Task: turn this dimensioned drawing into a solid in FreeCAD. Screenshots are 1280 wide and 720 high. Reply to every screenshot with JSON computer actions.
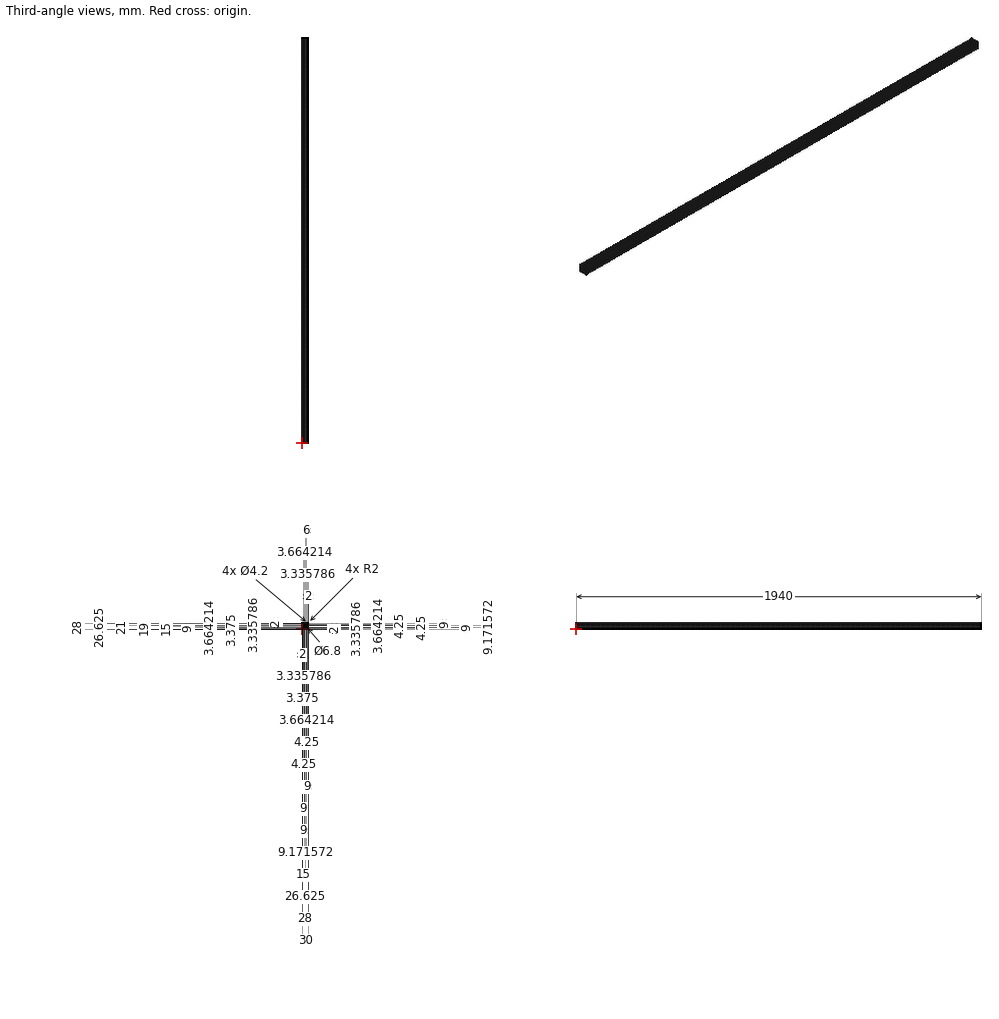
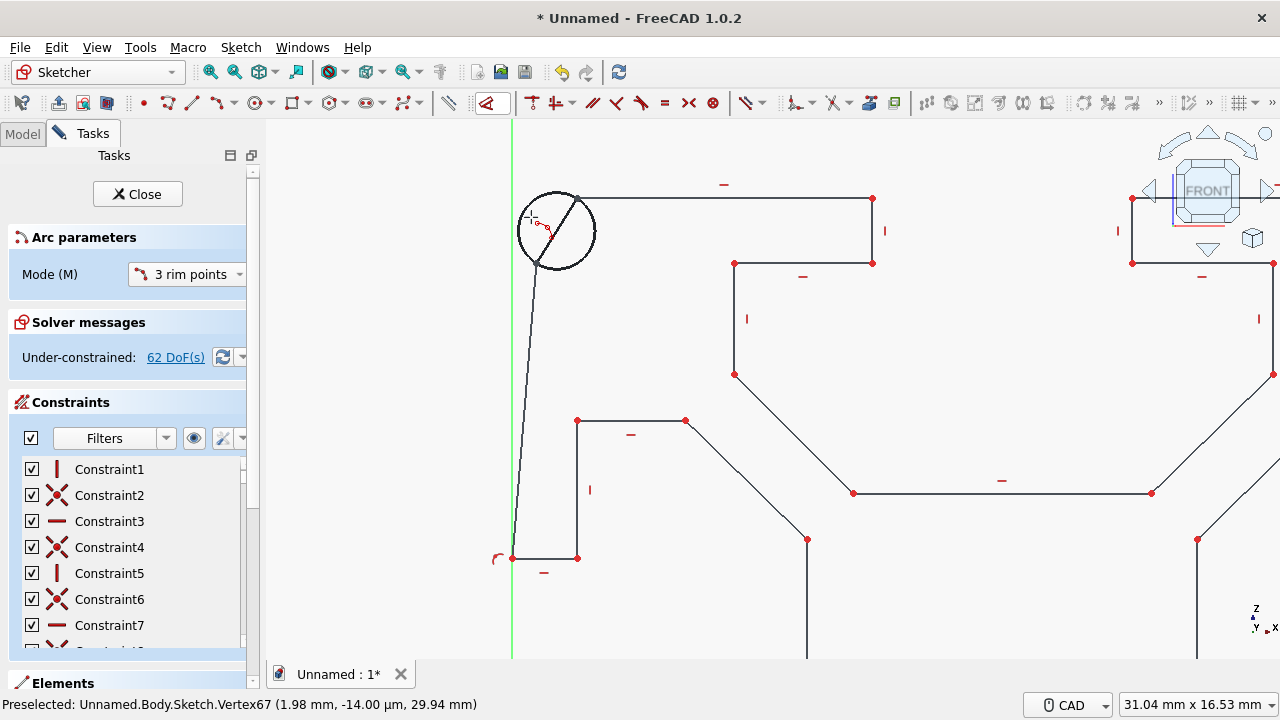
{"action": "left_click", "coordinate": [532, 216]}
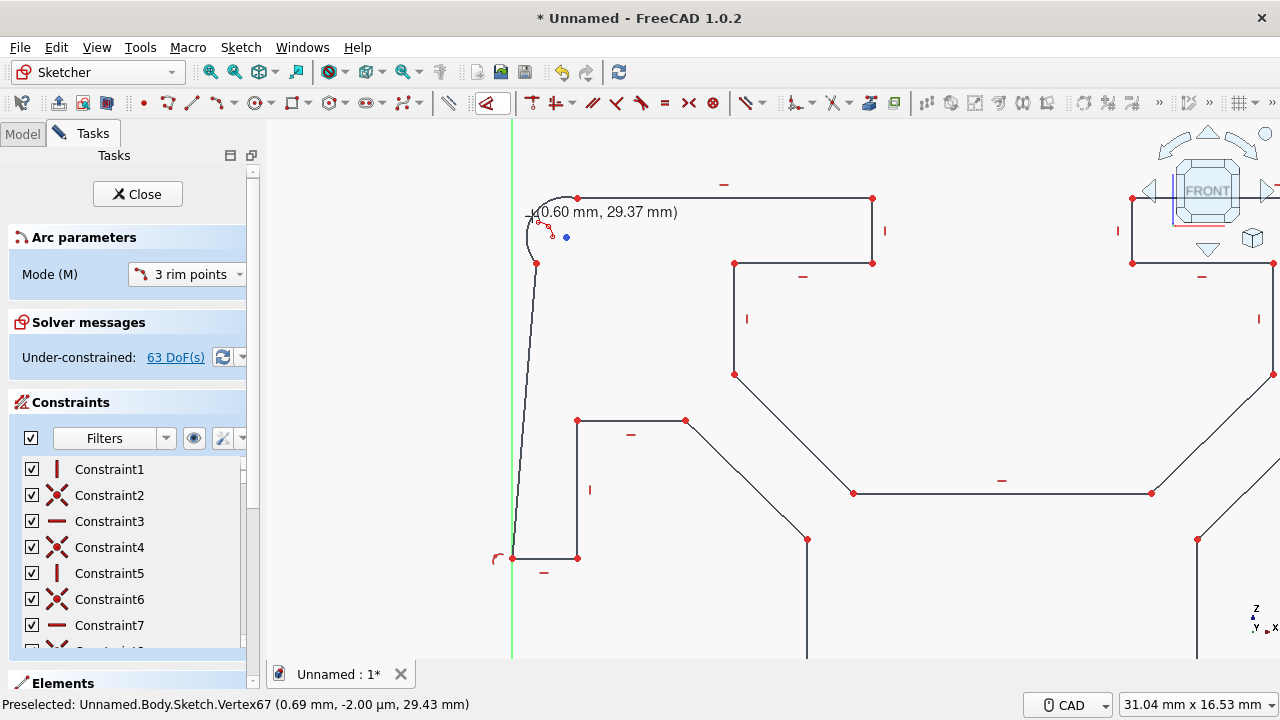
{"action": "scroll", "coordinate": [531, 216], "scroll_direction": "down", "scroll_amount": 5}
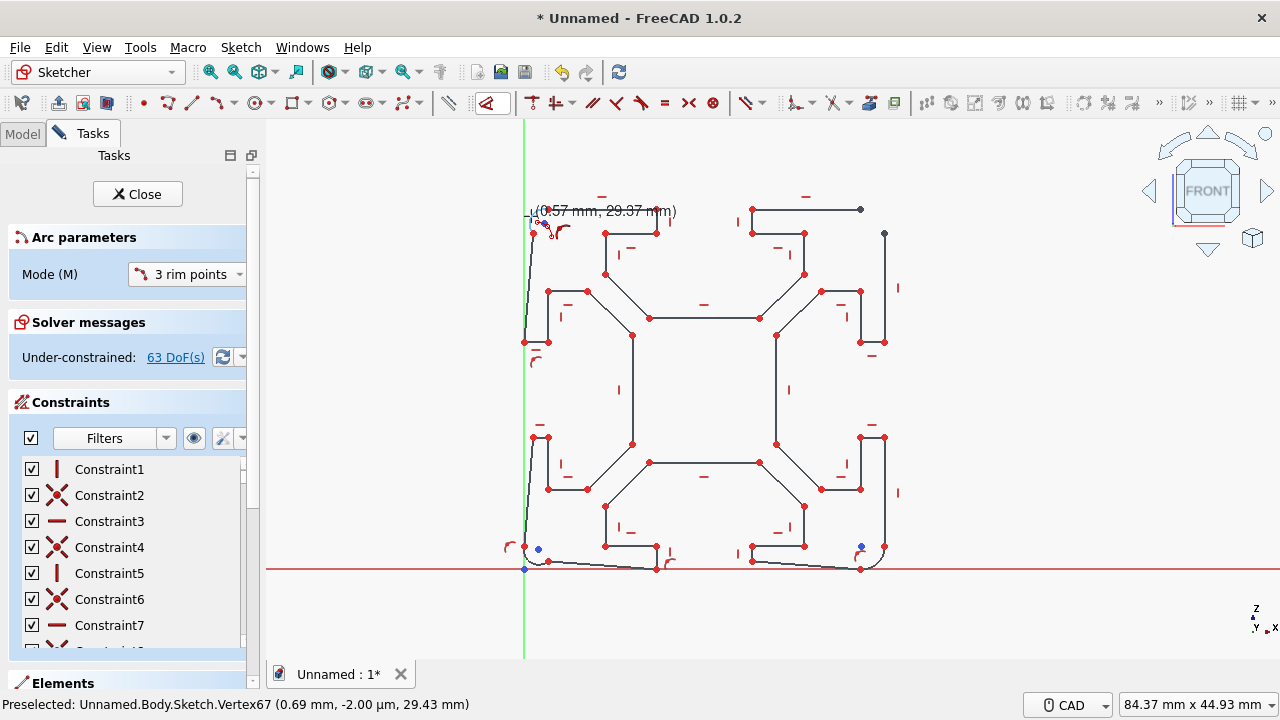
{"action": "left_click", "coordinate": [861, 210]}
{"action": "left_click", "coordinate": [885, 234]}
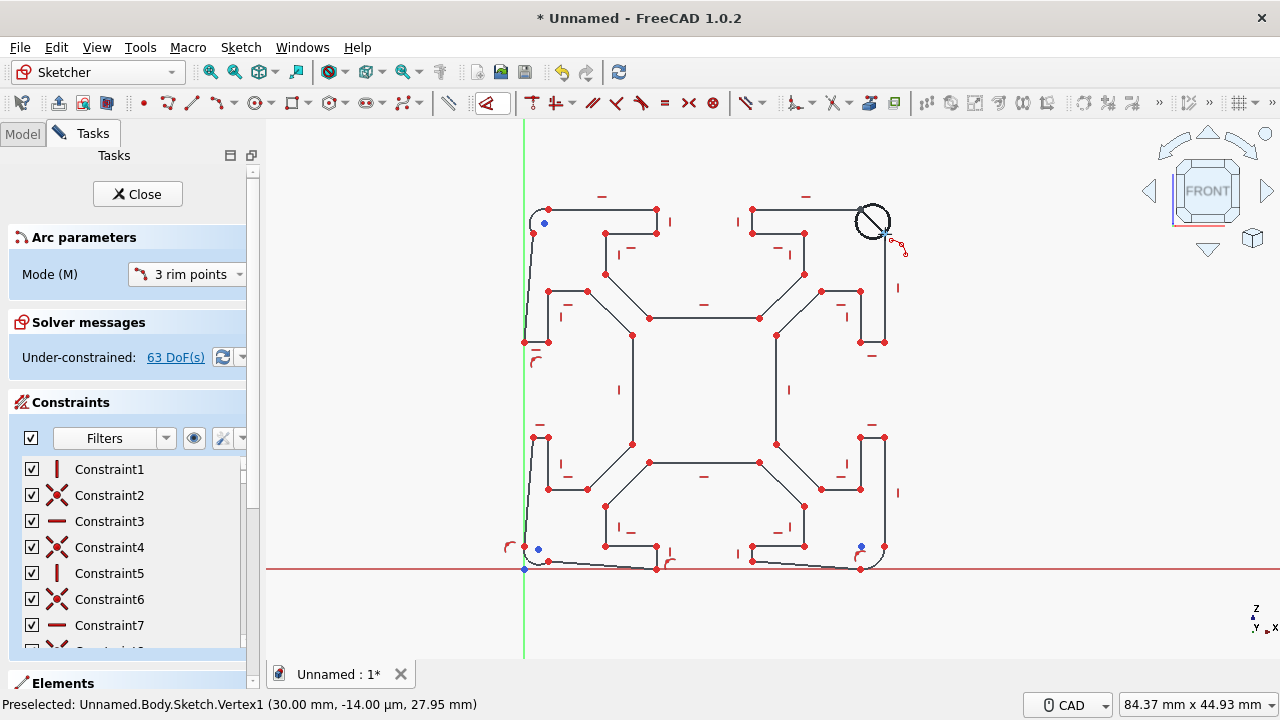
{"action": "scroll", "coordinate": [878, 216], "scroll_direction": "up", "scroll_amount": 5}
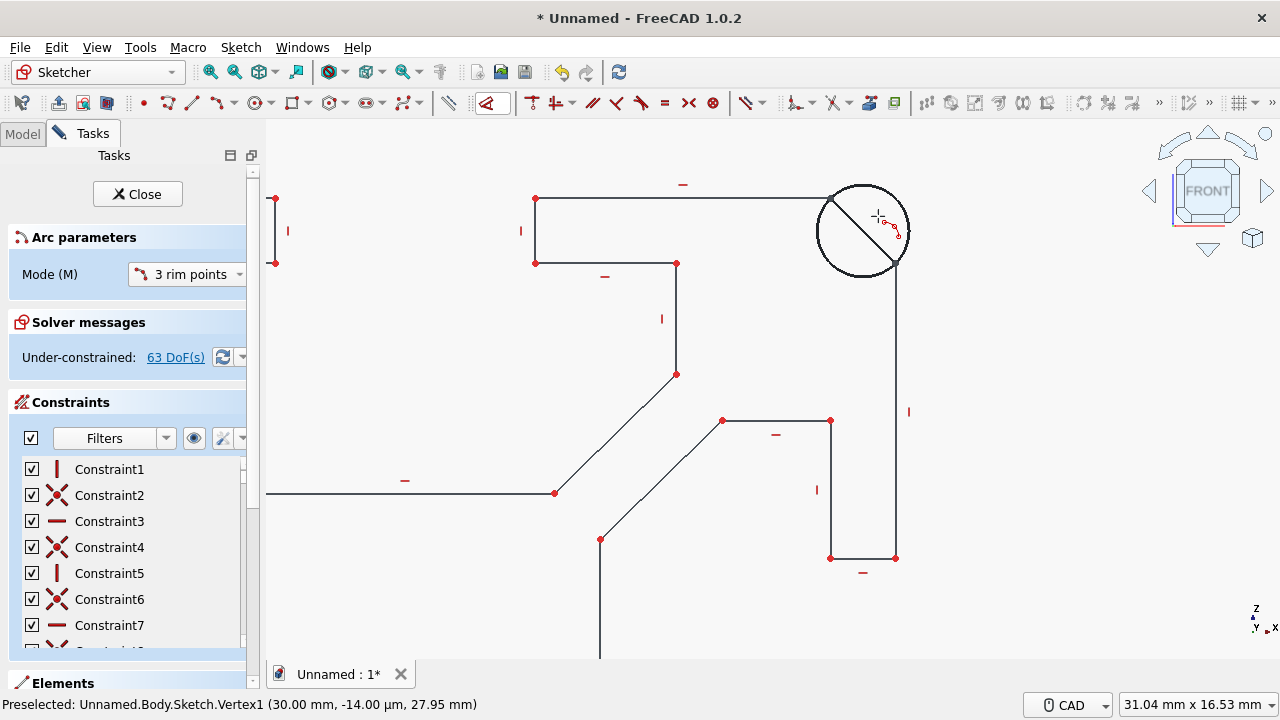
{"action": "left_click", "coordinate": [876, 216]}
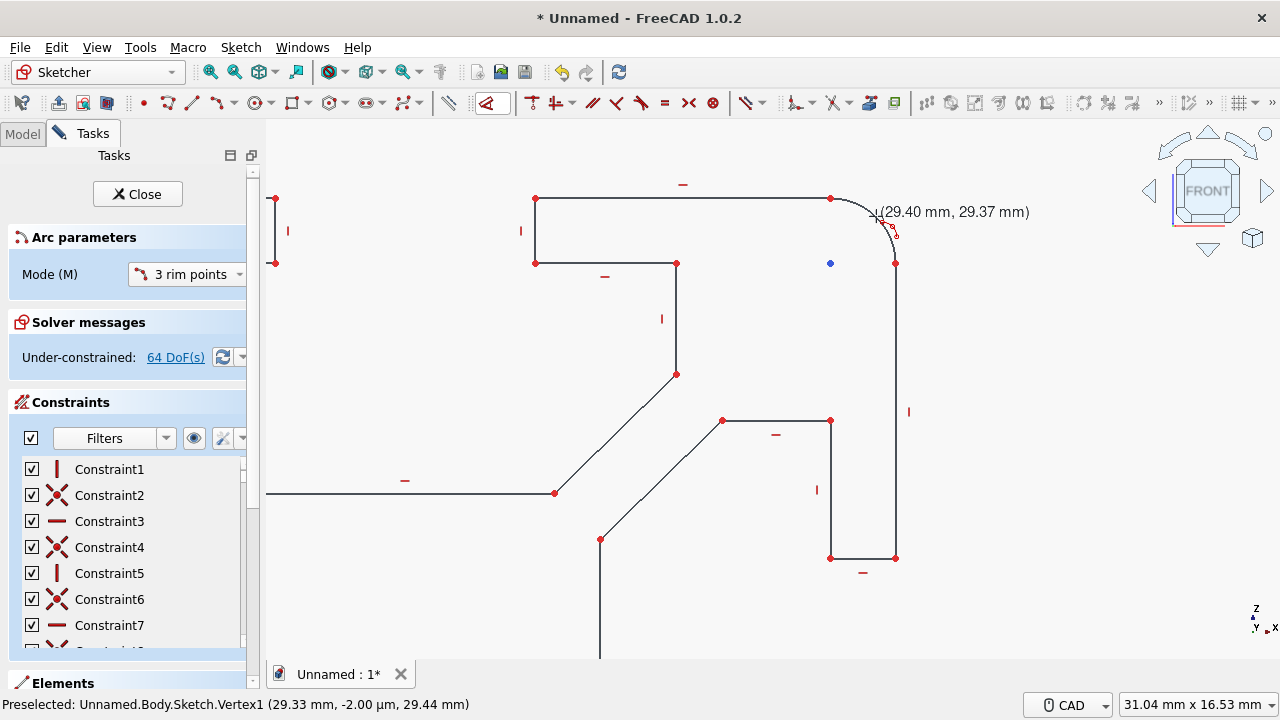
{"action": "left_click", "coordinate": [256, 104]}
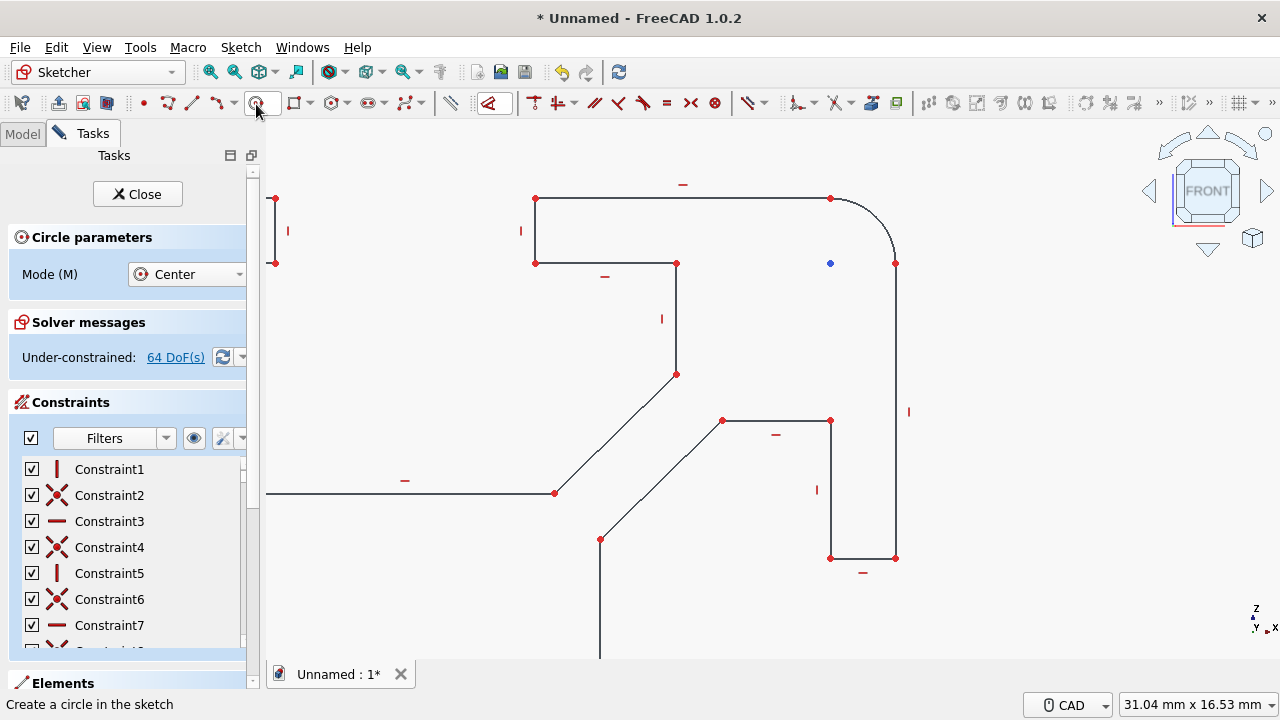
{"action": "left_click", "coordinate": [785, 307]}
{"action": "mouse_move", "coordinate": [737, 258]}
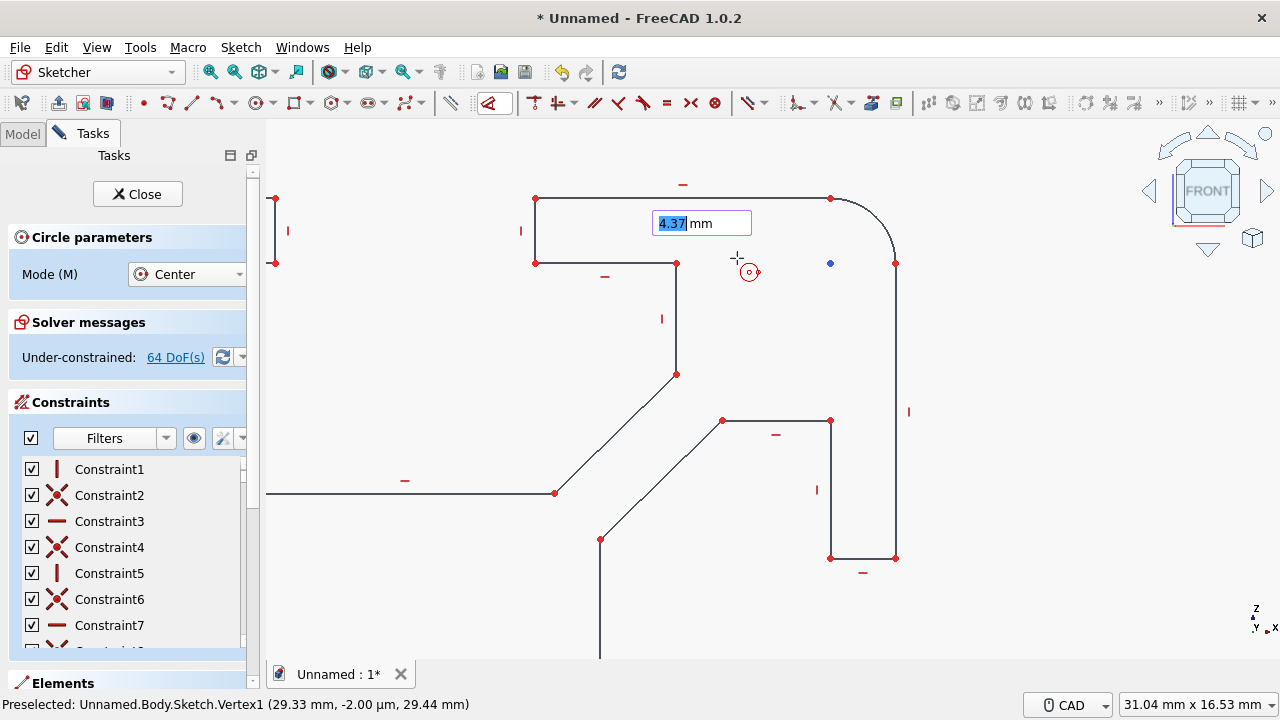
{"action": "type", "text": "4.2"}
{"action": "key", "text": "Return"}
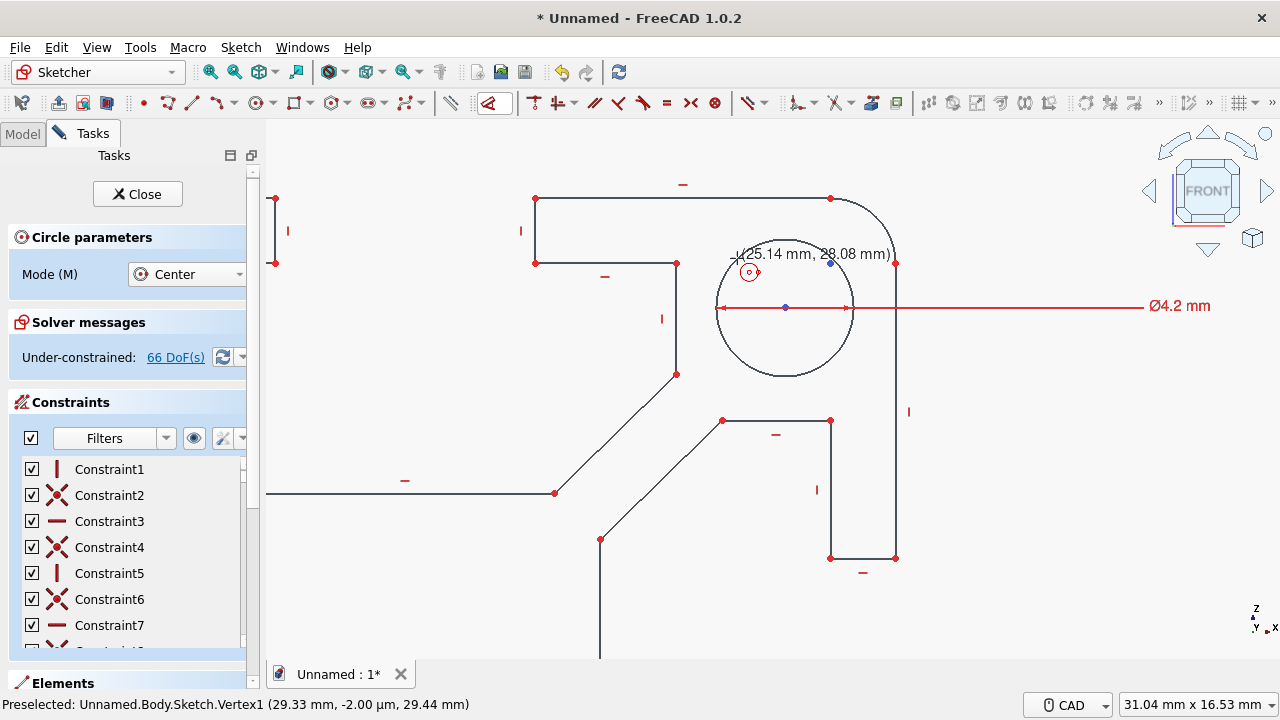
{"action": "scroll", "coordinate": [878, 216], "scroll_direction": "down", "scroll_amount": 5}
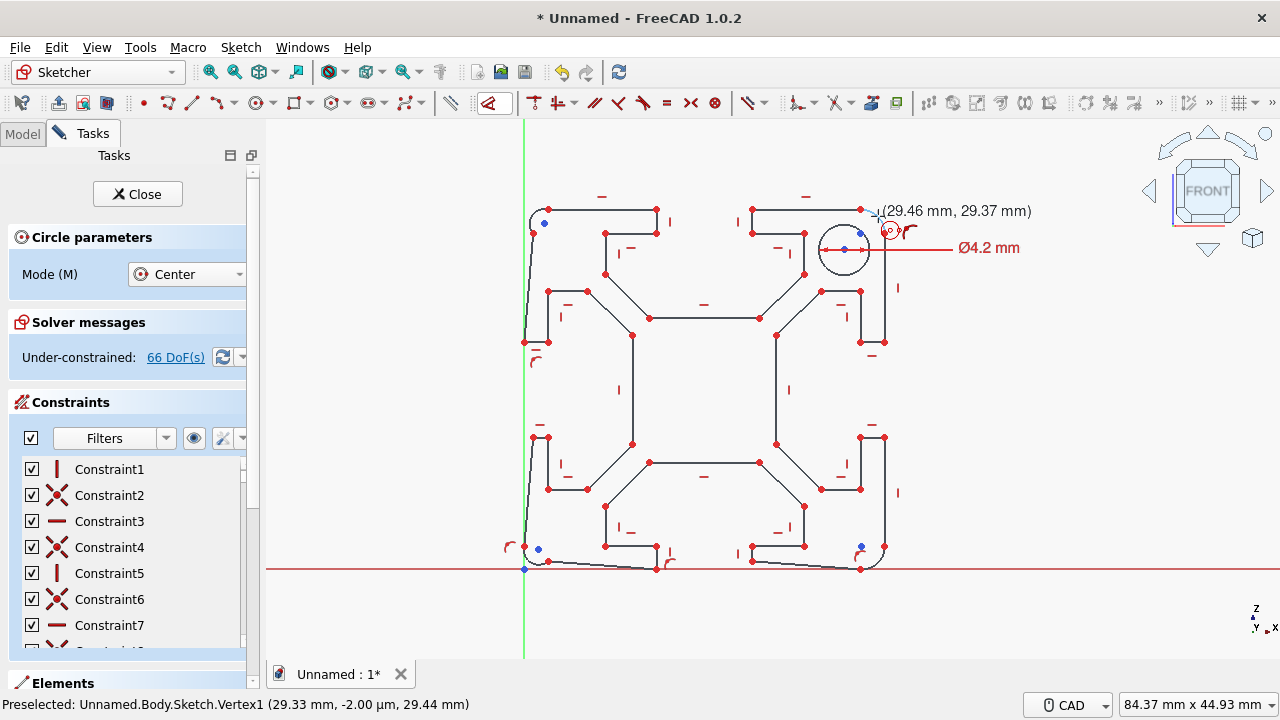
{"action": "left_click", "coordinate": [565, 249]}
{"action": "mouse_move", "coordinate": [583, 232]}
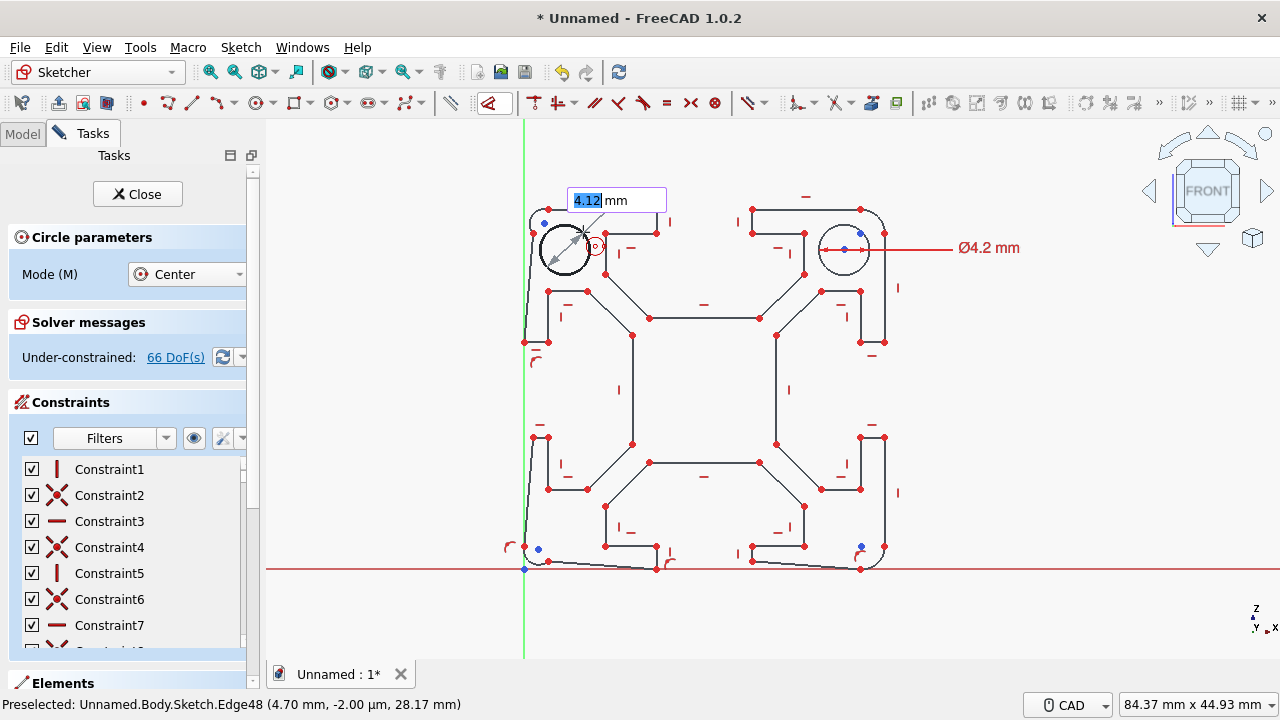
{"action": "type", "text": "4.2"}
{"action": "key", "text": "Return"}